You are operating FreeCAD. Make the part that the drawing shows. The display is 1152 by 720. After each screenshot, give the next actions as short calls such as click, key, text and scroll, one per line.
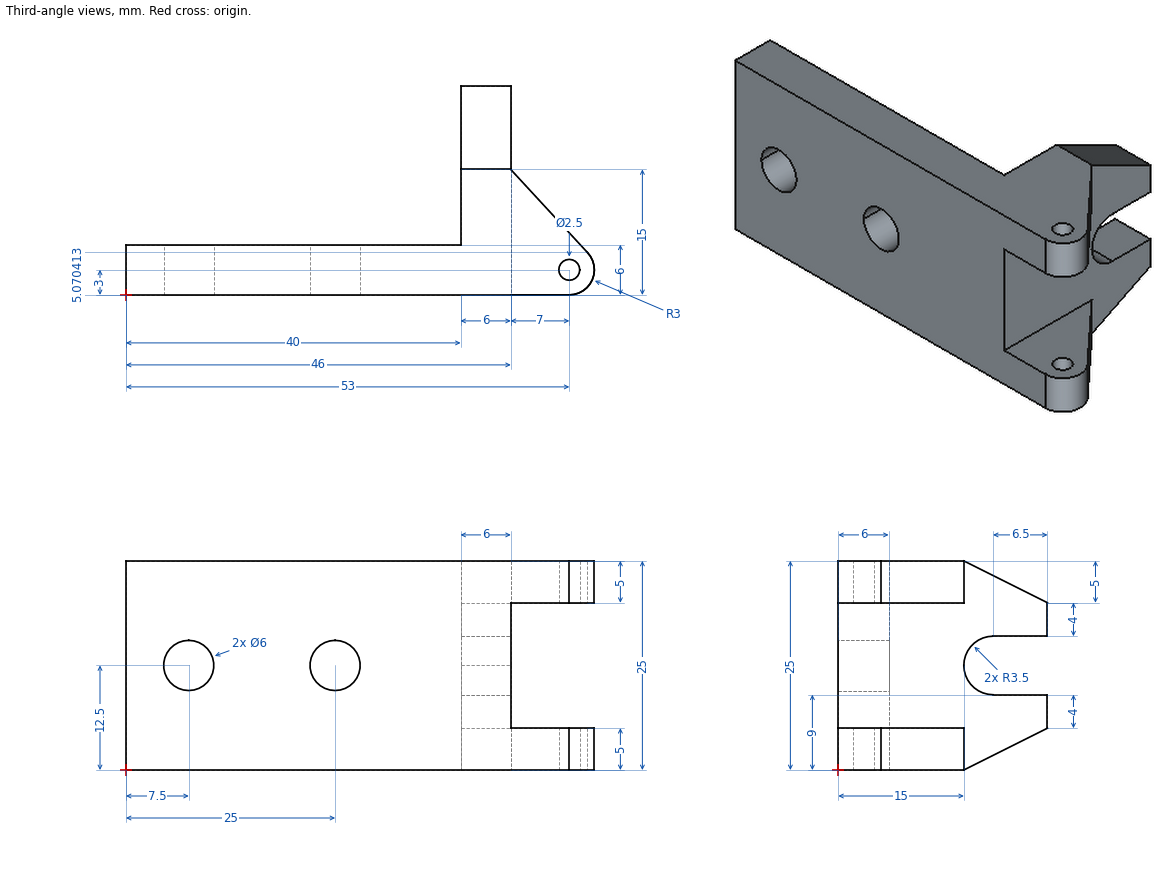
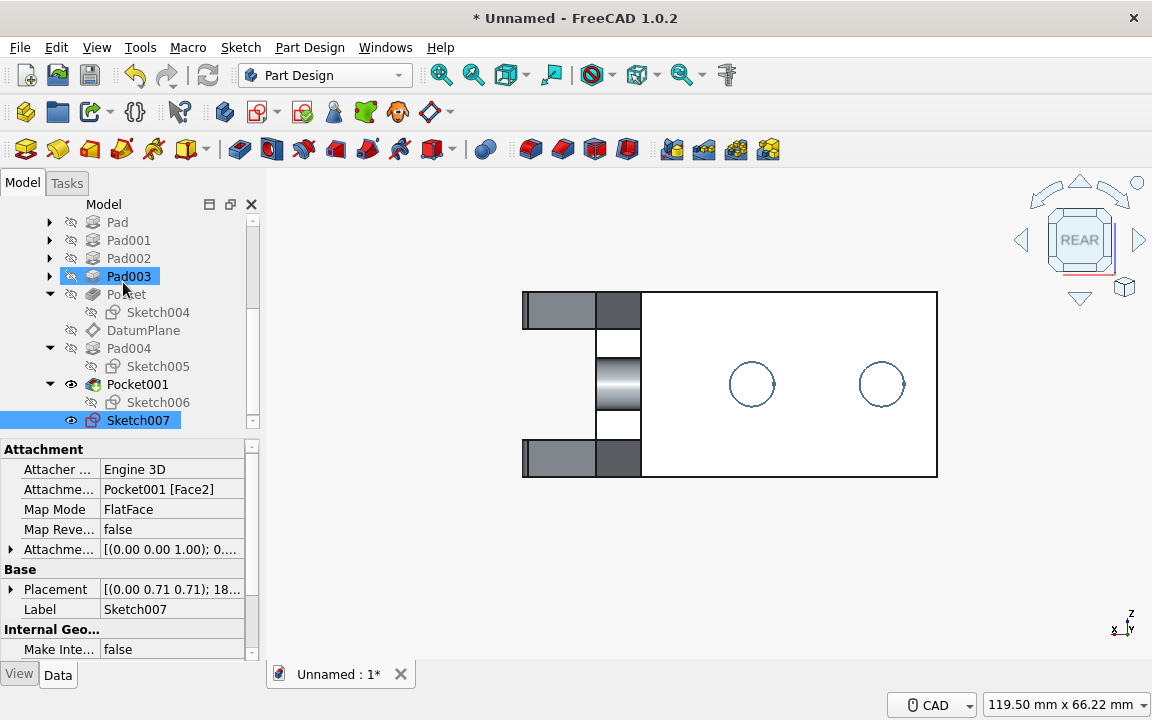
click(240, 150)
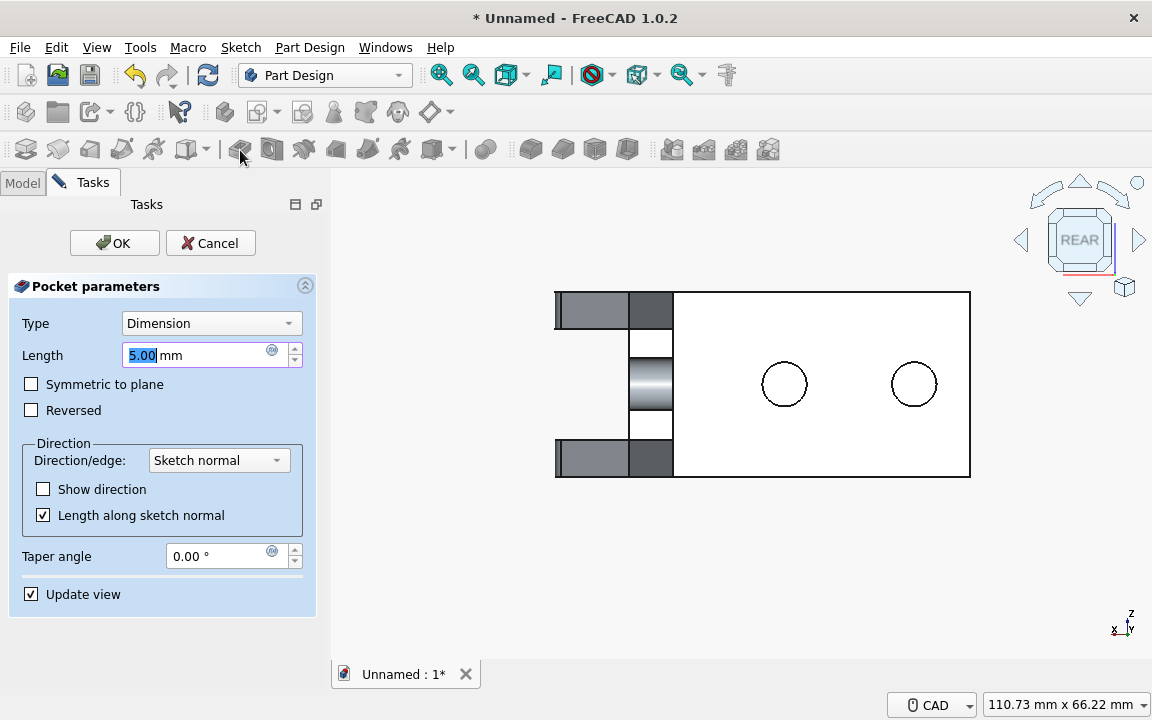
text(6)
key(Tab)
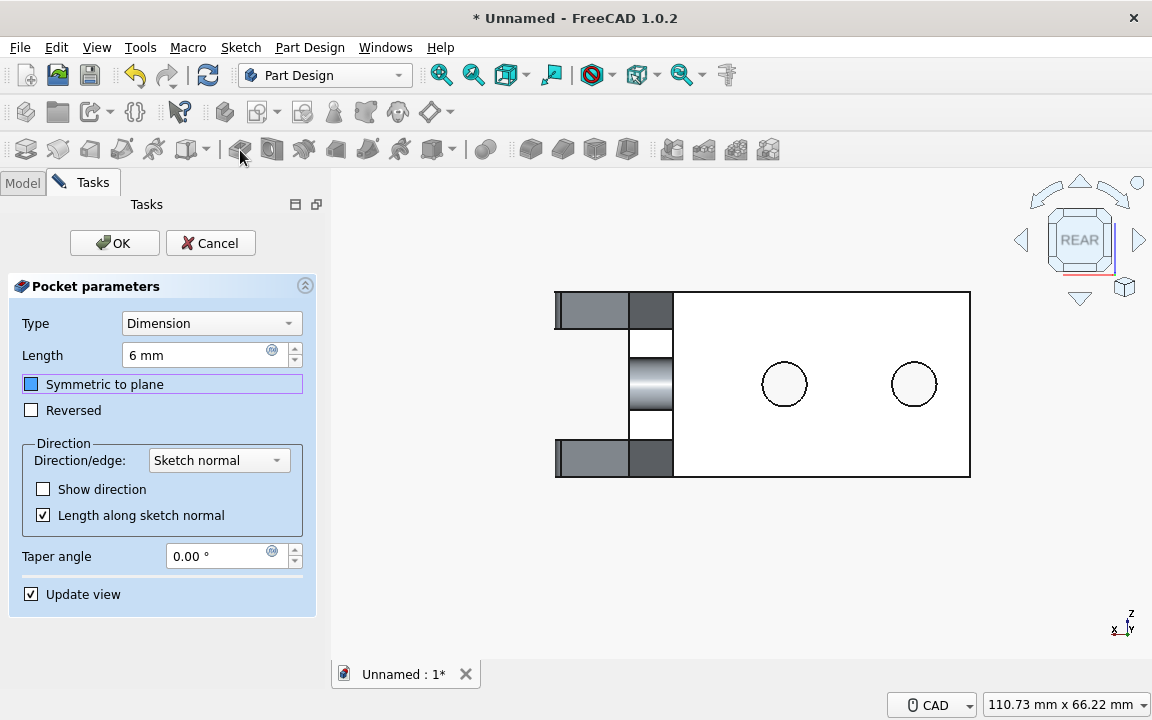
click(115, 243)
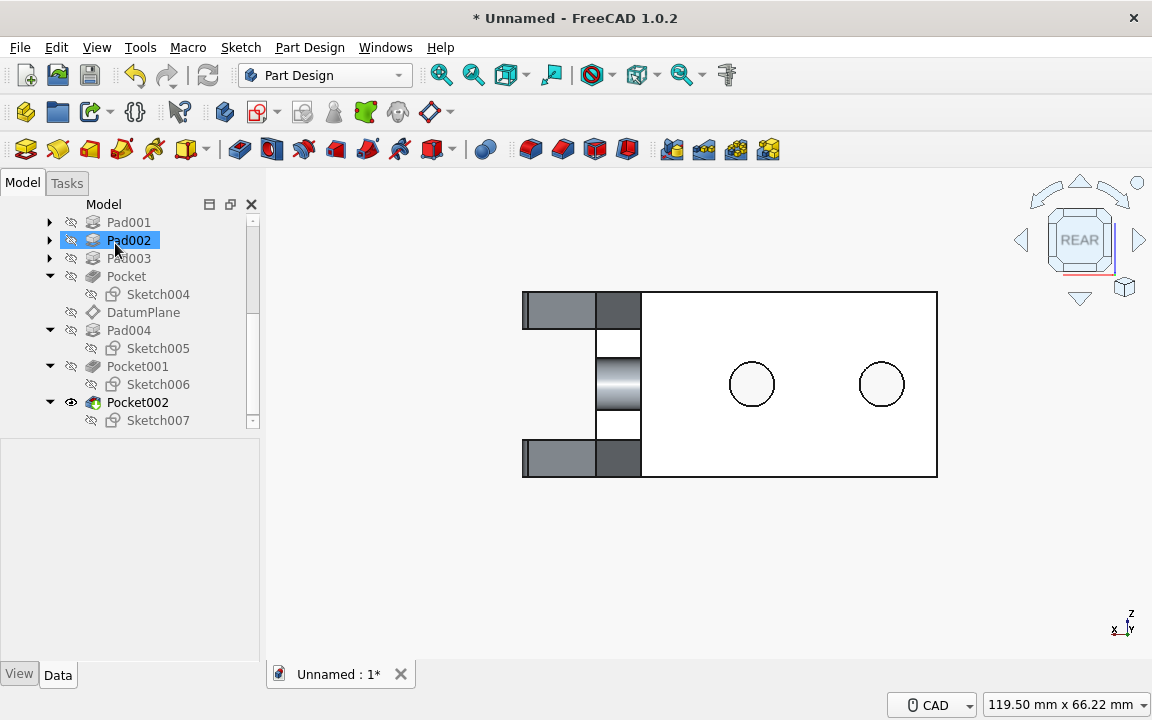
key(0)